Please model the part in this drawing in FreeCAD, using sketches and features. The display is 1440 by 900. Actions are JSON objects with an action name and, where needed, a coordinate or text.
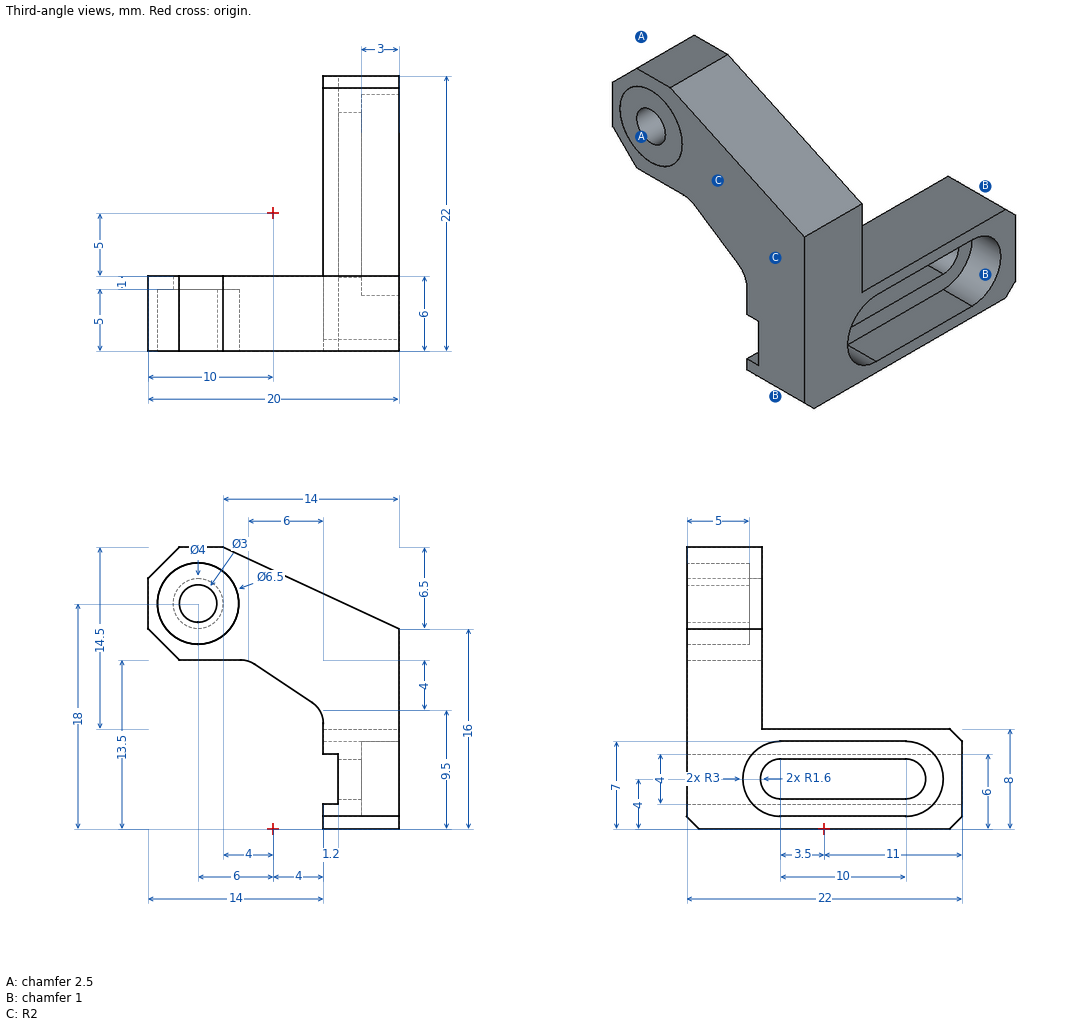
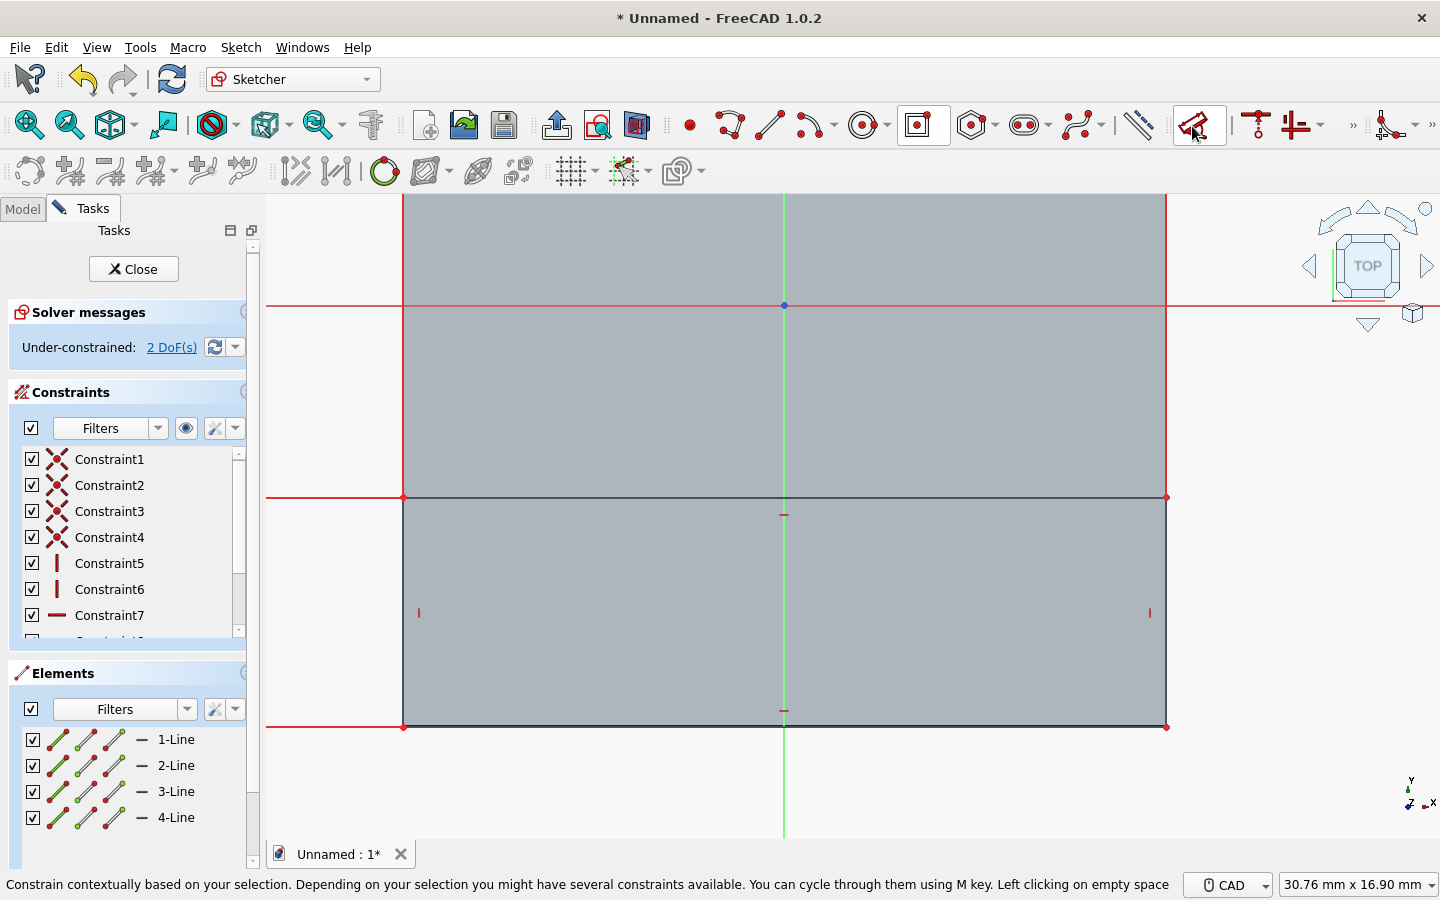
{"action": "left_click", "coordinate": [403, 498]}
{"action": "left_click", "coordinate": [369, 402]}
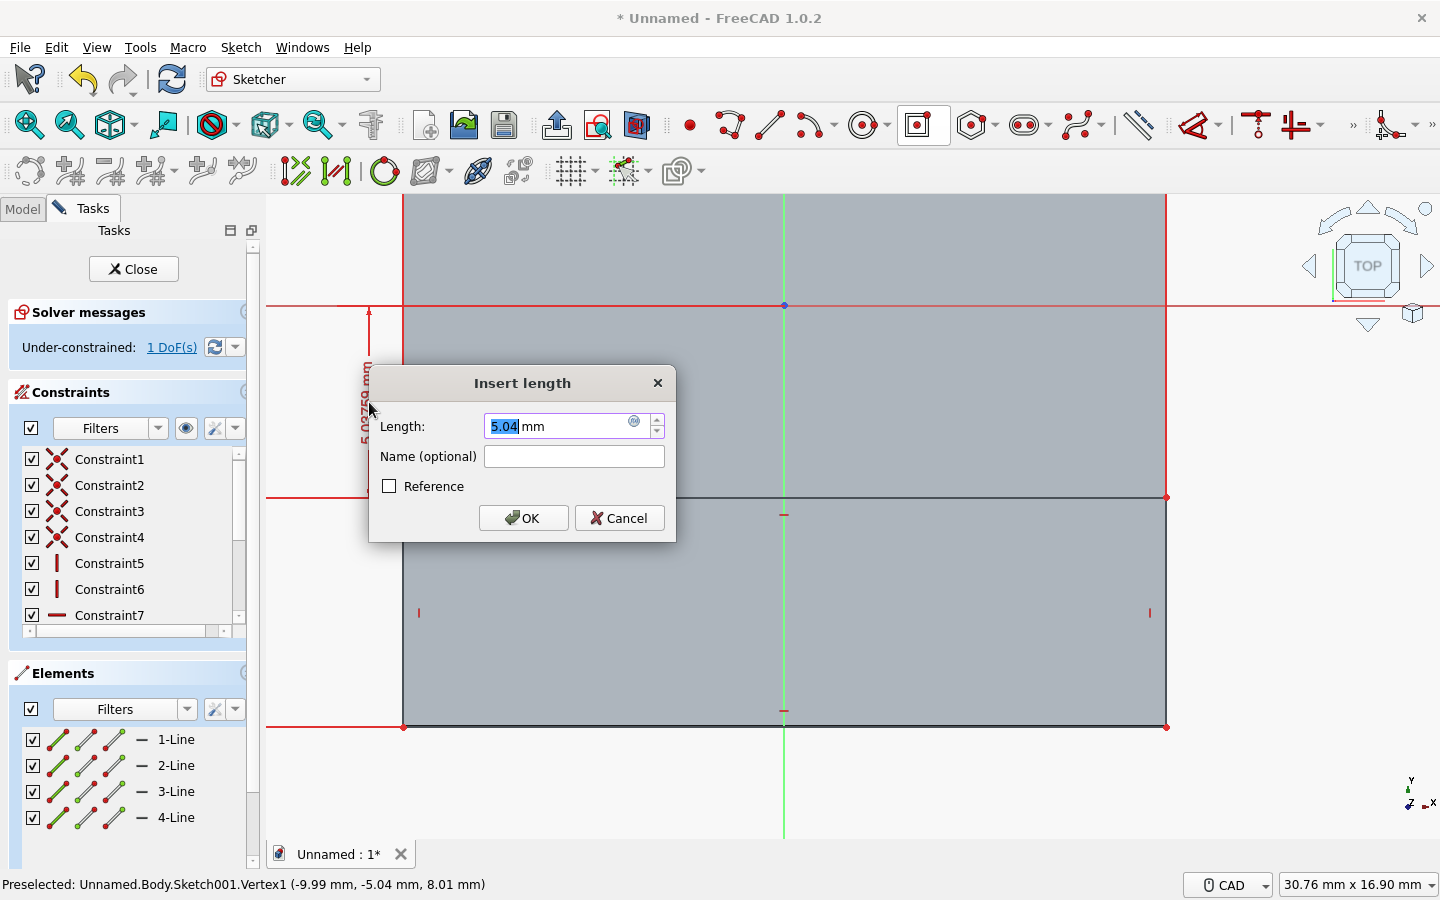
{"action": "type", "text": "5"}
{"action": "key", "text": "Return"}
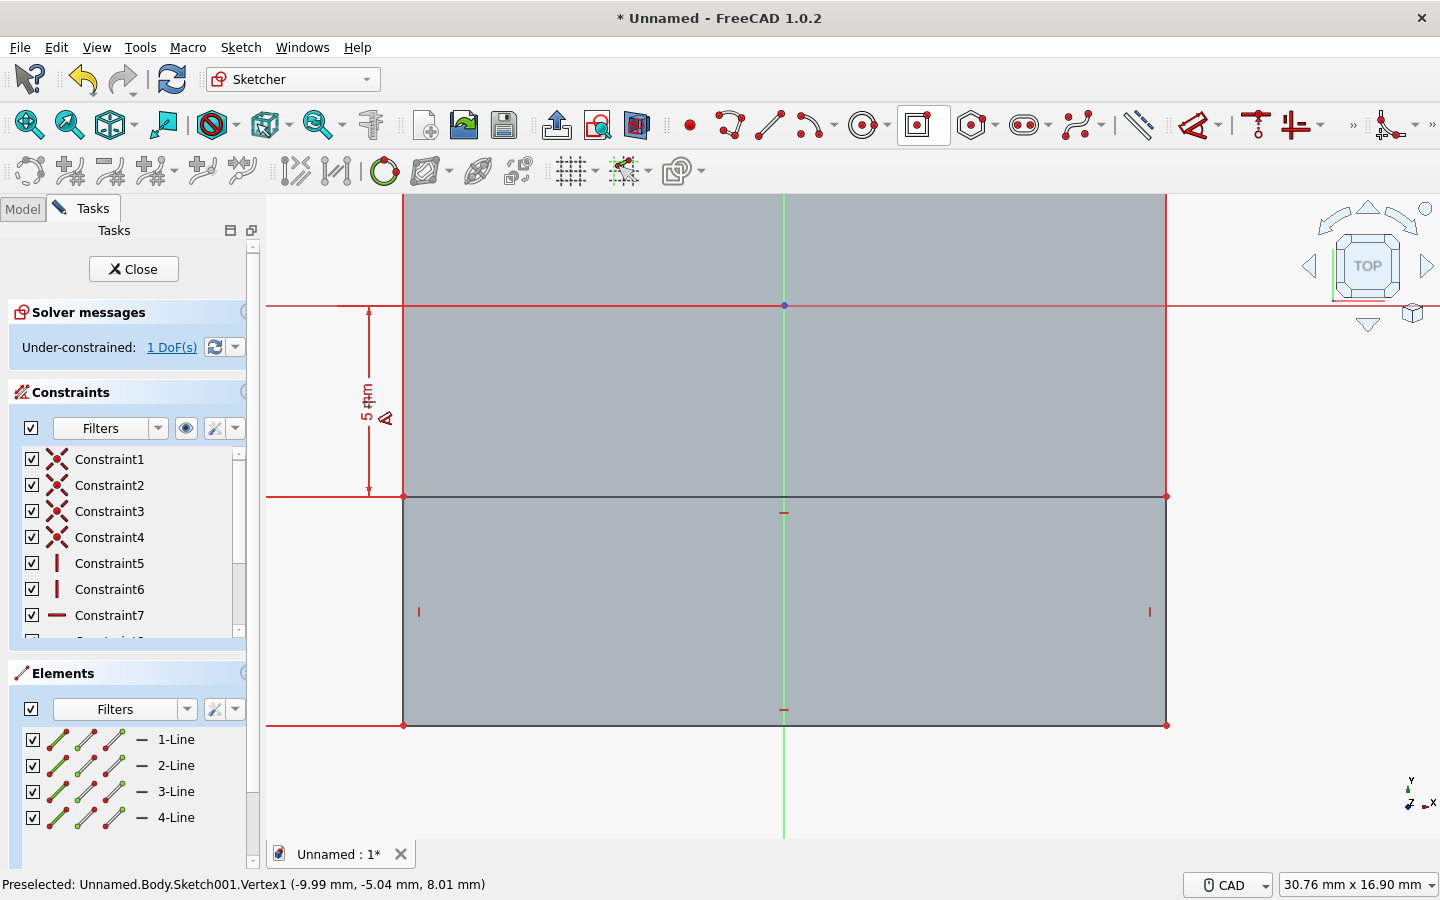
{"action": "left_click", "coordinate": [403, 497]}
{"action": "left_click", "coordinate": [594, 272]}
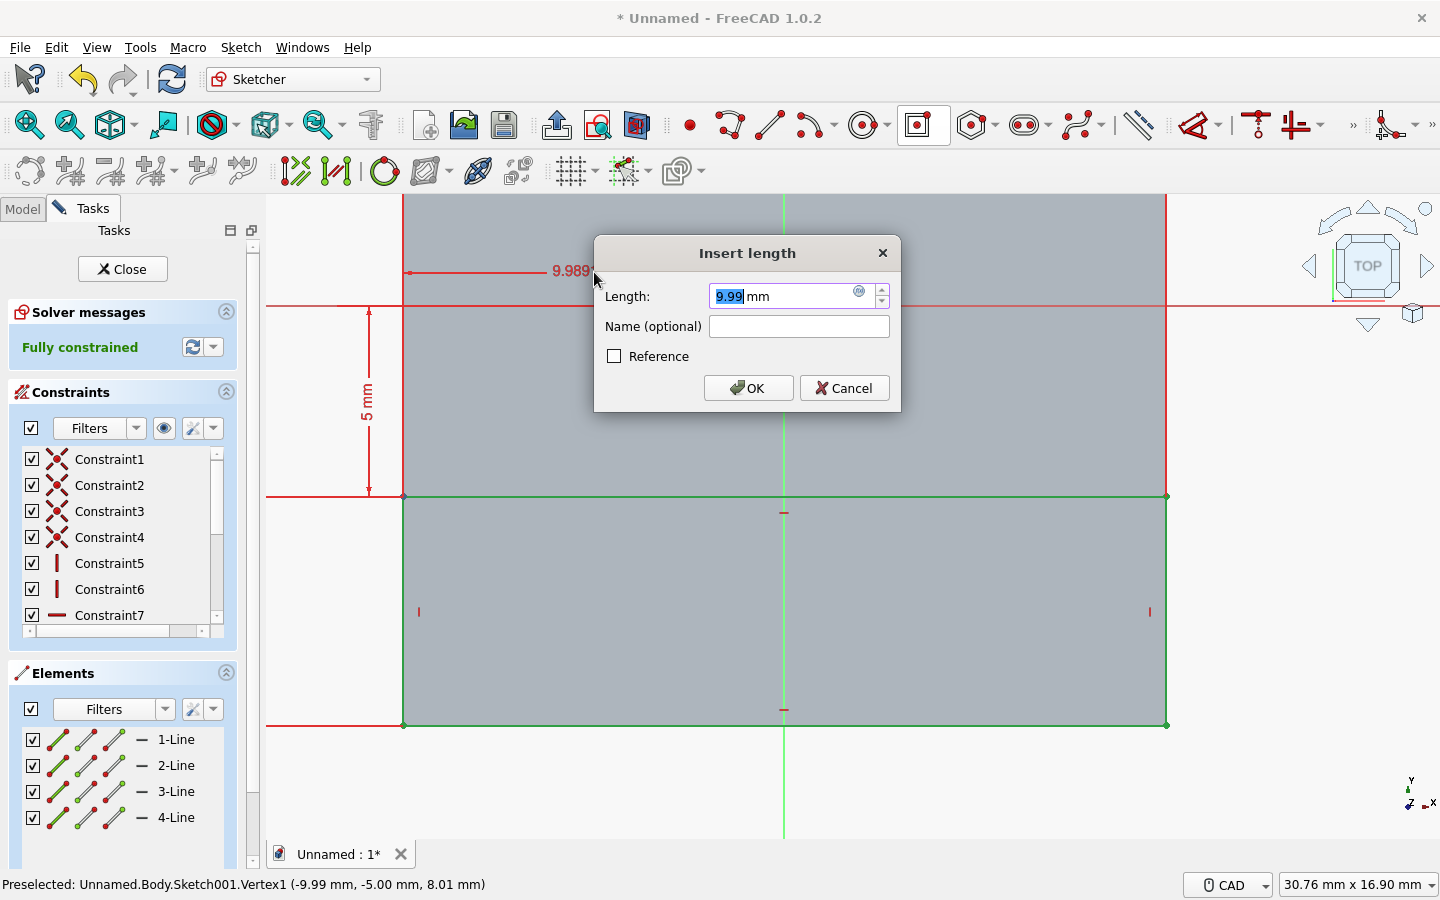
{"action": "type", "text": "10"}
{"action": "key", "text": "Return"}
{"action": "key", "text": "Escape"}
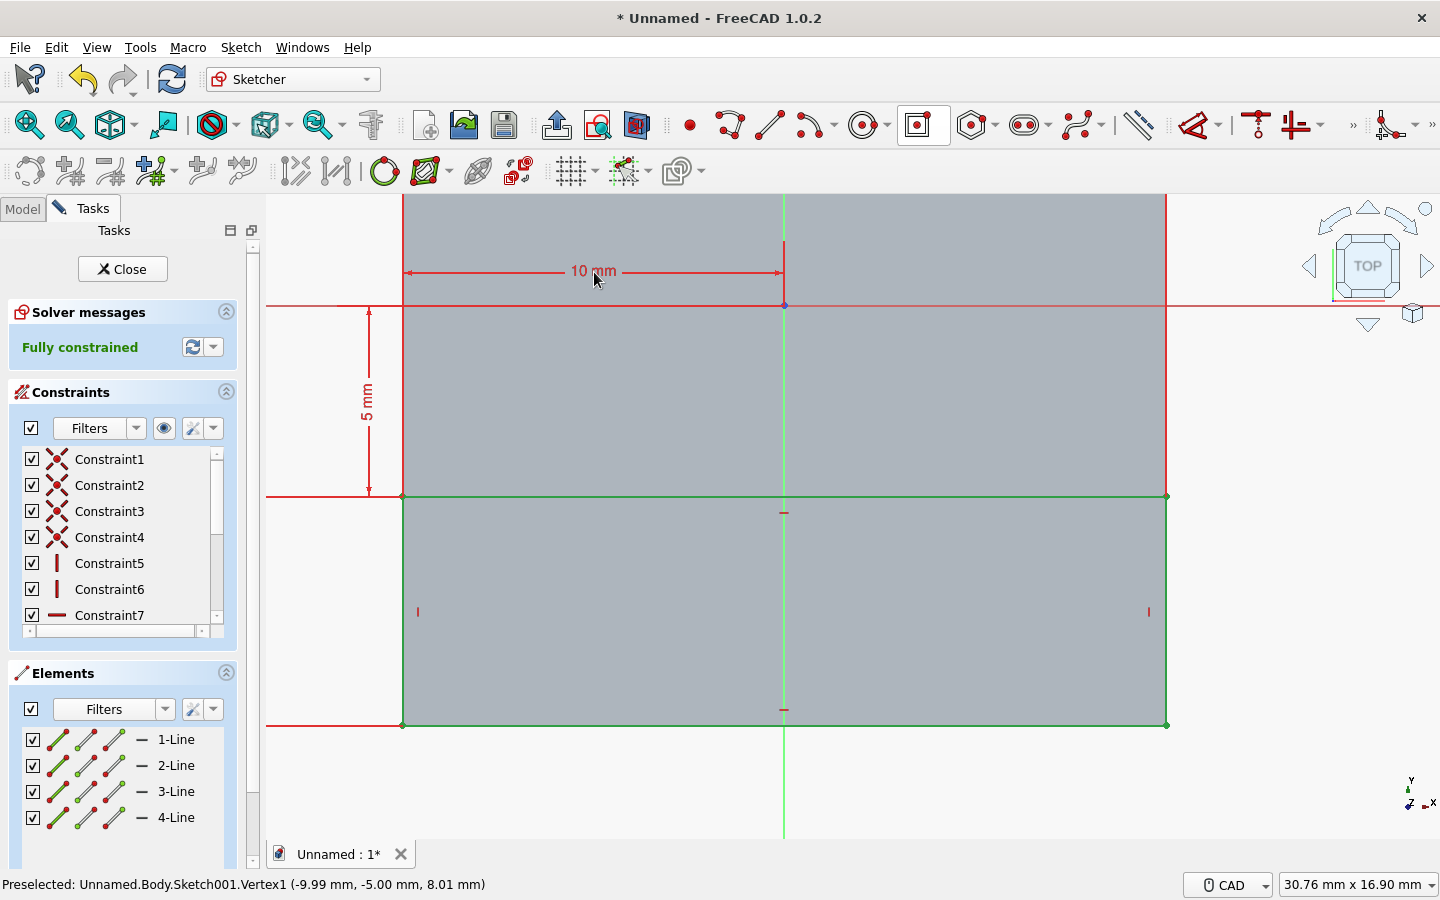
{"action": "left_click", "coordinate": [123, 269]}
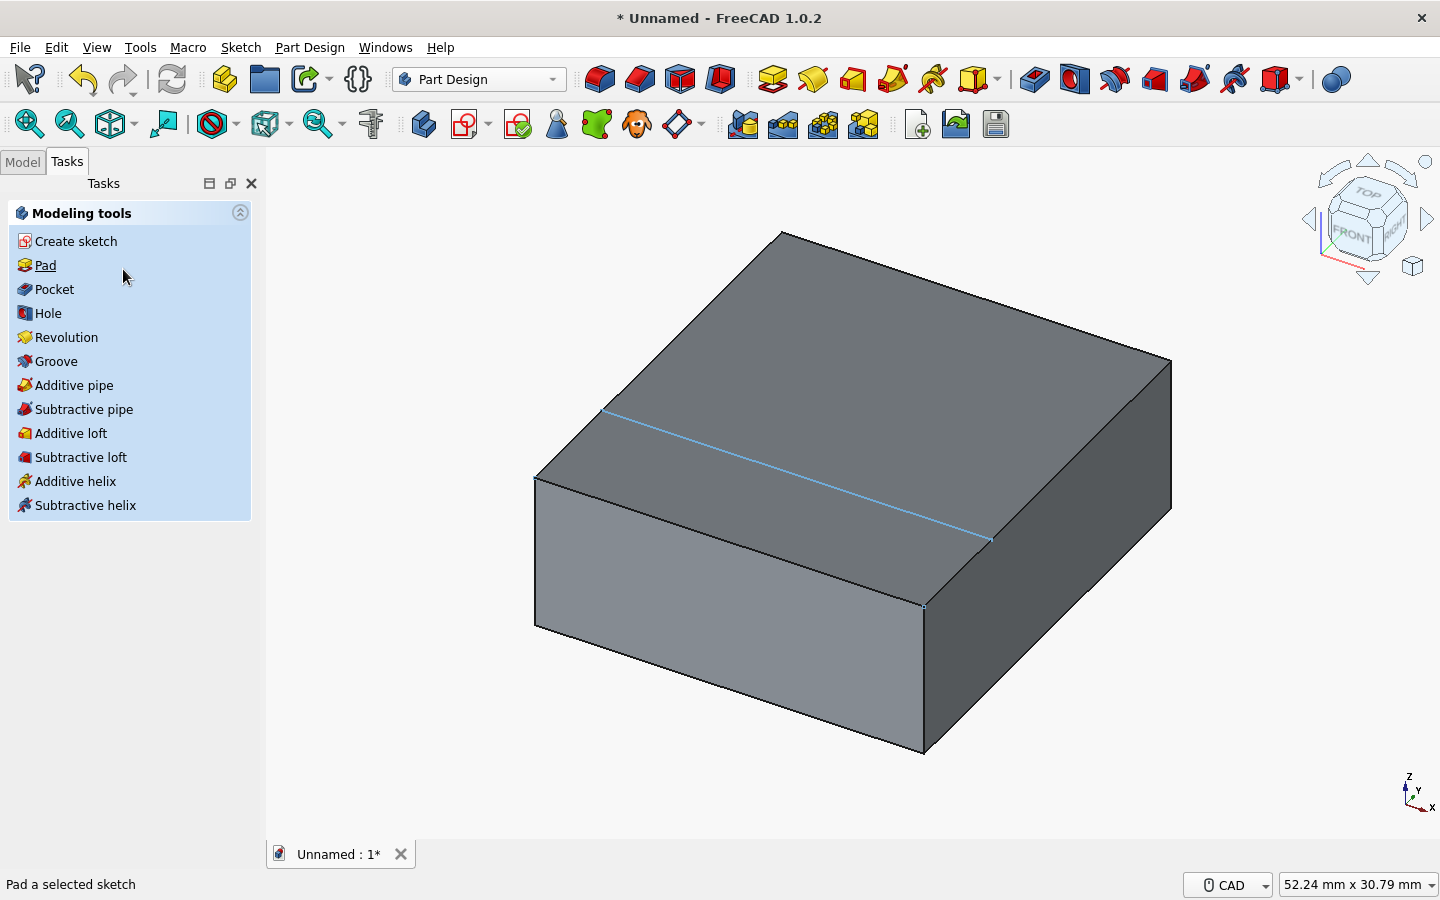
{"action": "left_click", "coordinate": [774, 80]}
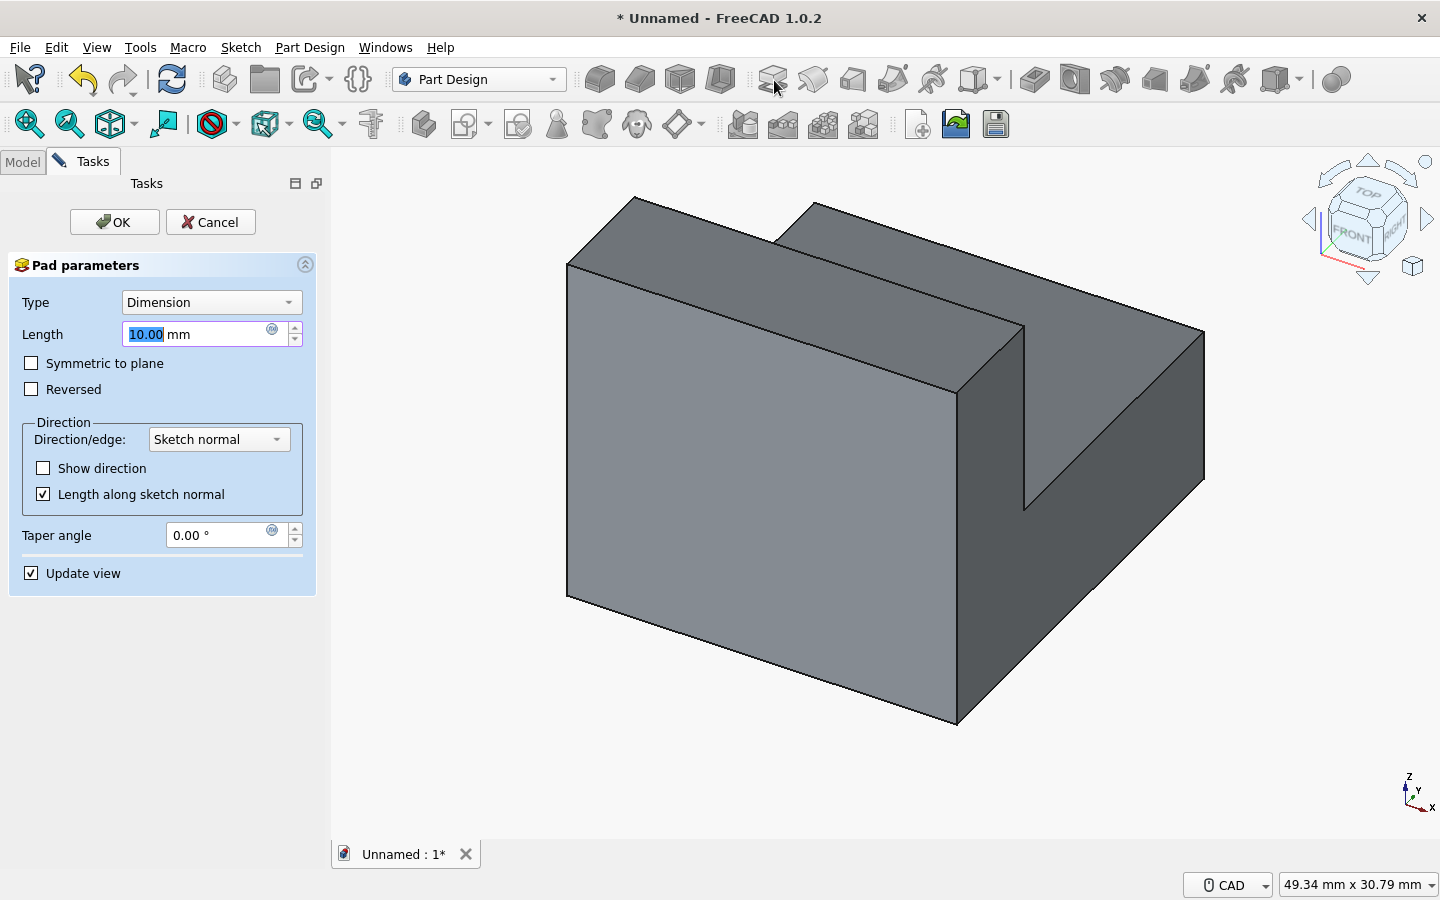
{"action": "type", "text": "14.5"}
{"action": "key", "text": "Tab"}